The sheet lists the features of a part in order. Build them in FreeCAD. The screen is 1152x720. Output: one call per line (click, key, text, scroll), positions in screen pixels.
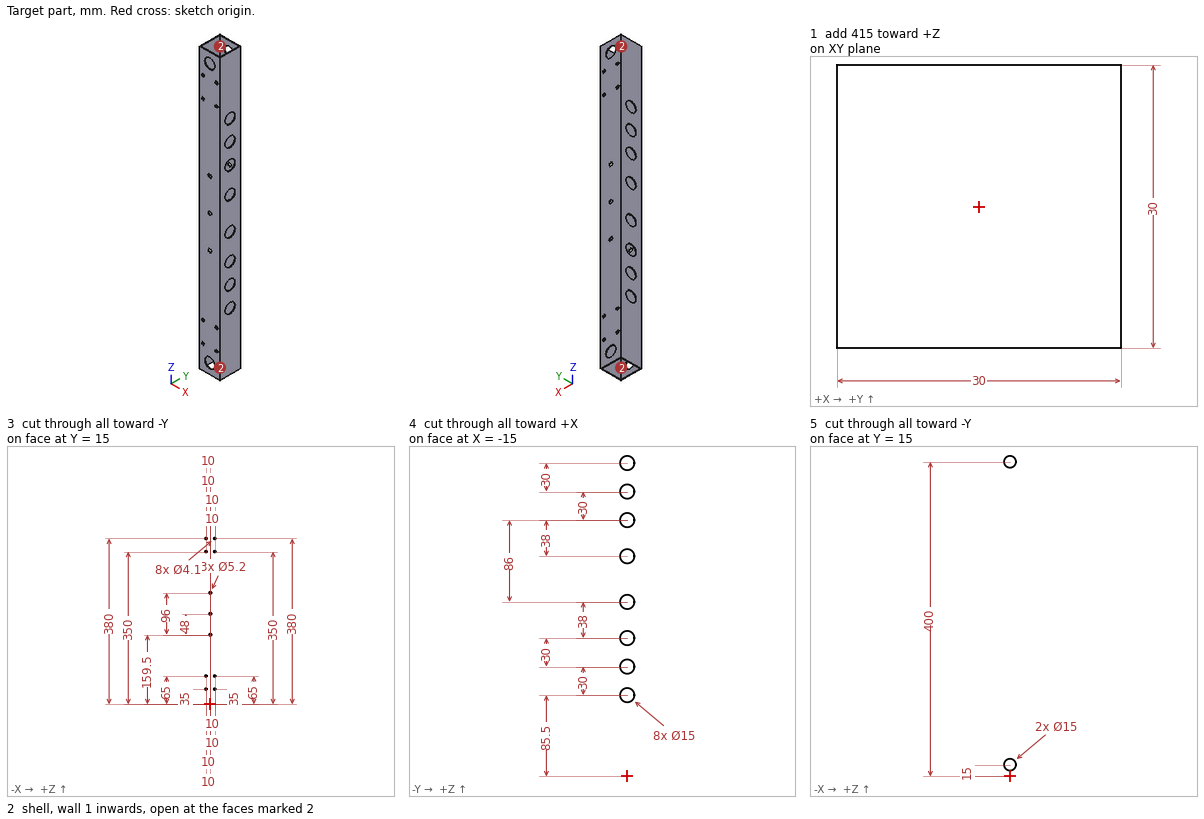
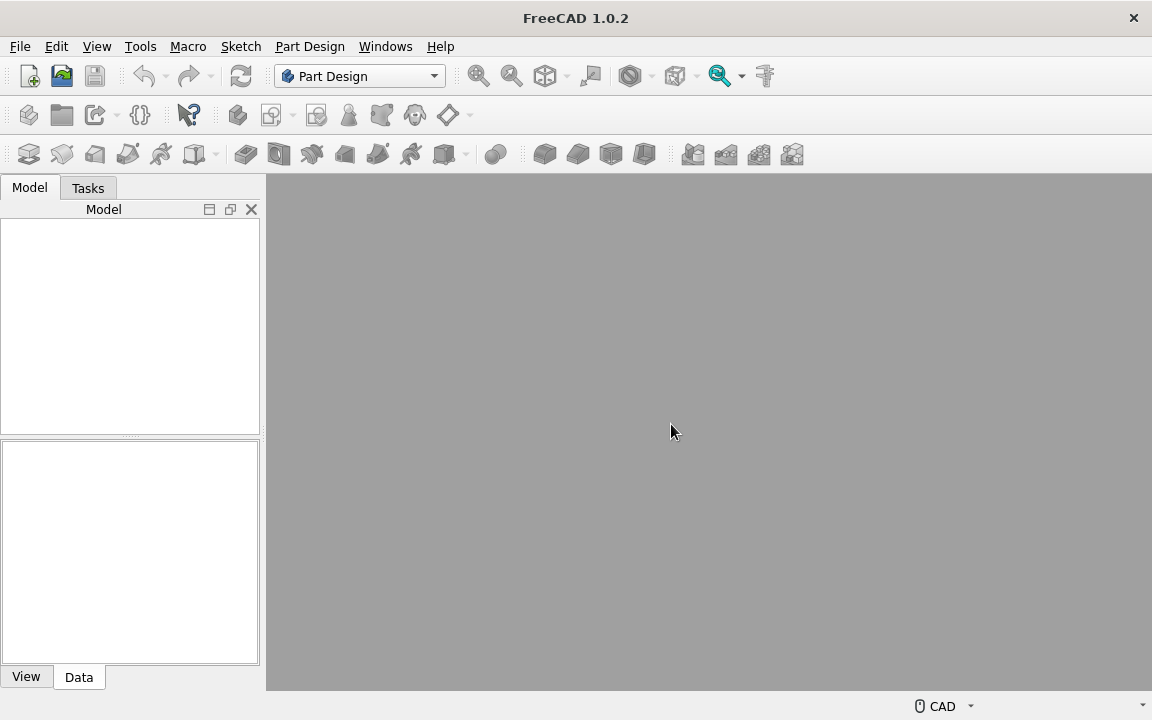
key(ctrl+n)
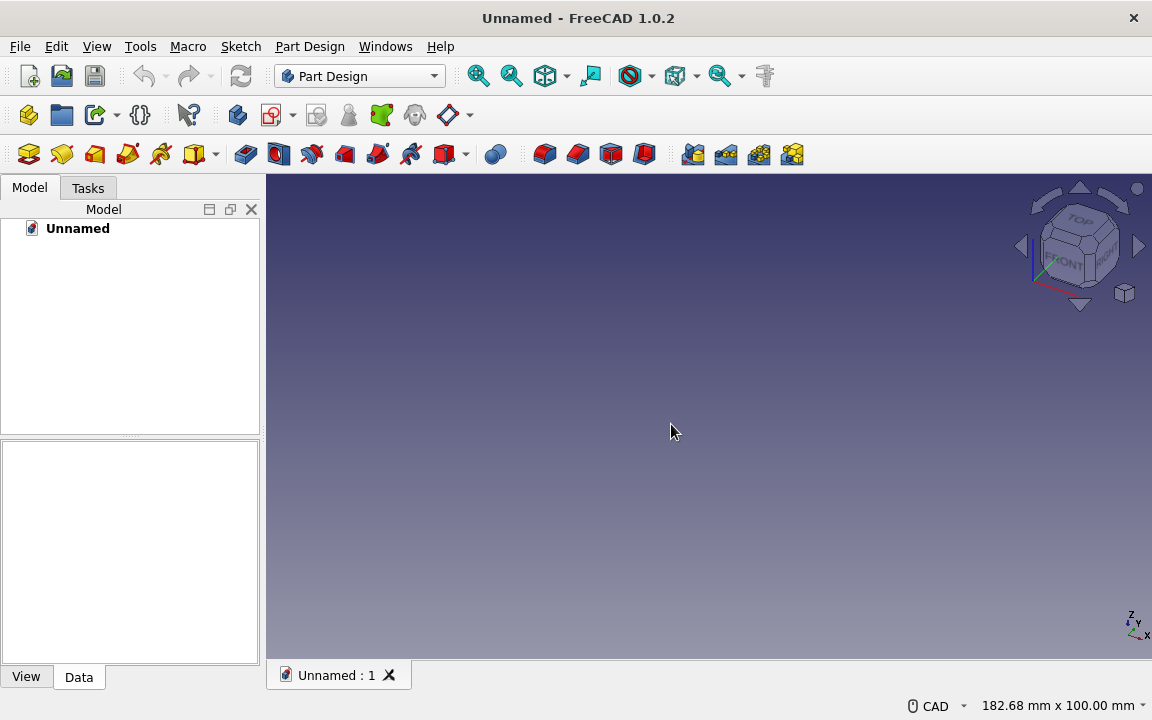
click(270, 116)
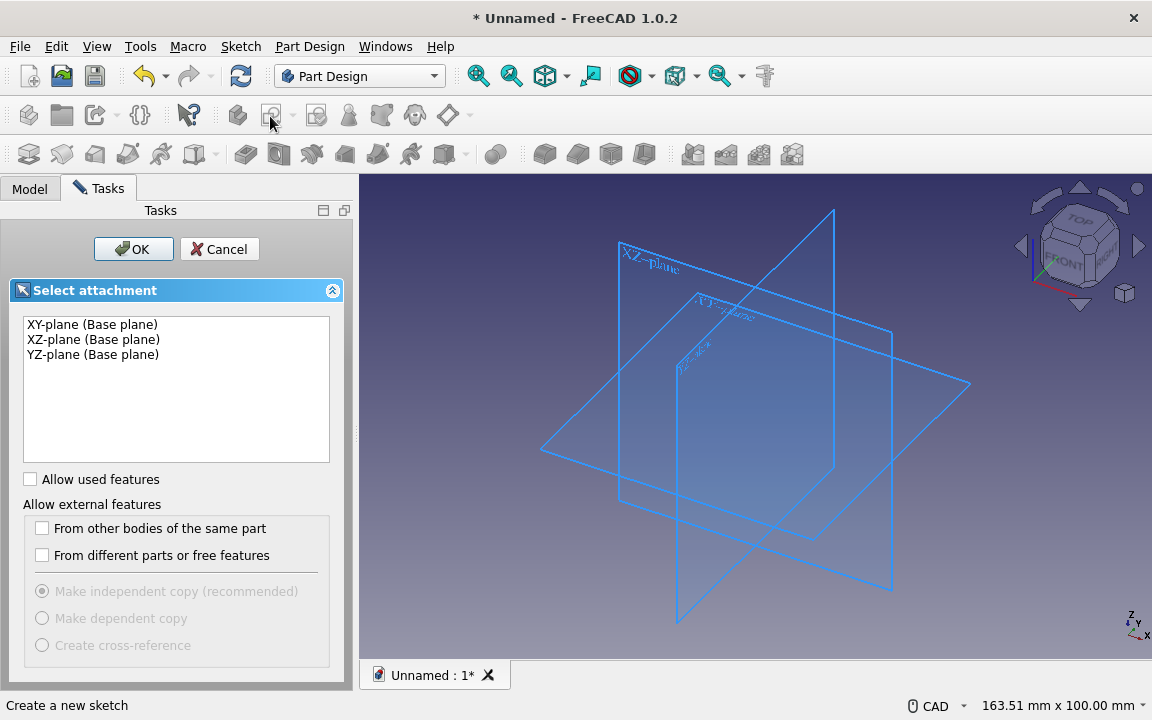
click(84, 324)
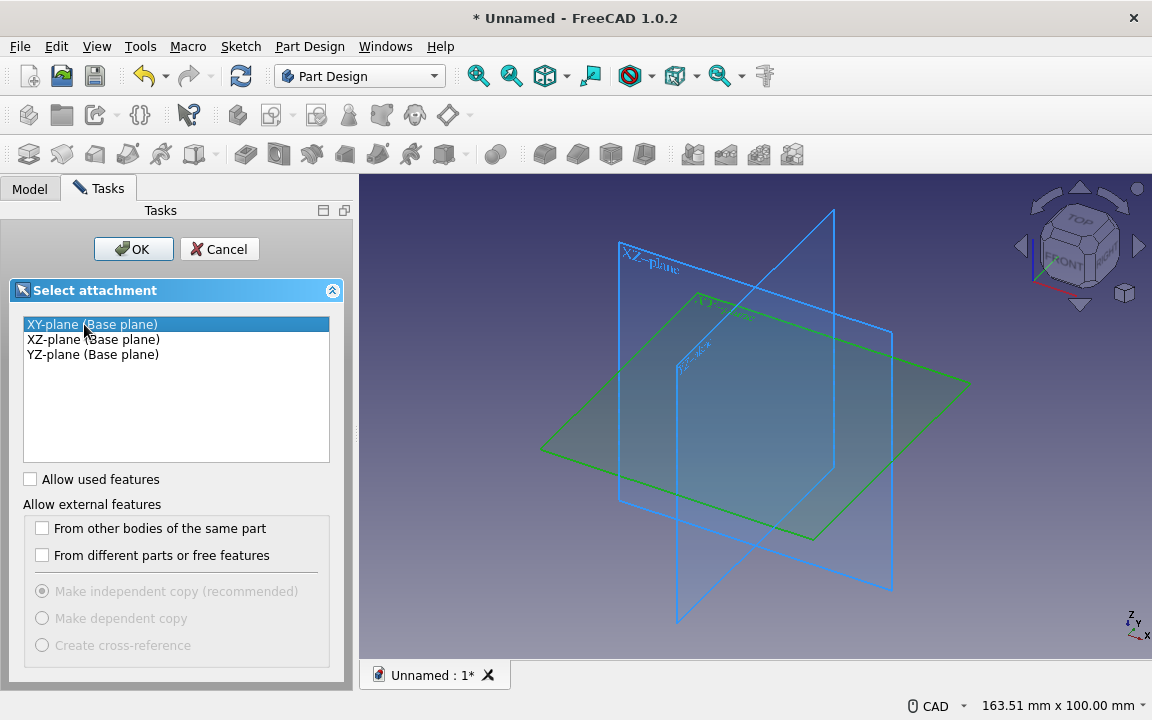
click(134, 249)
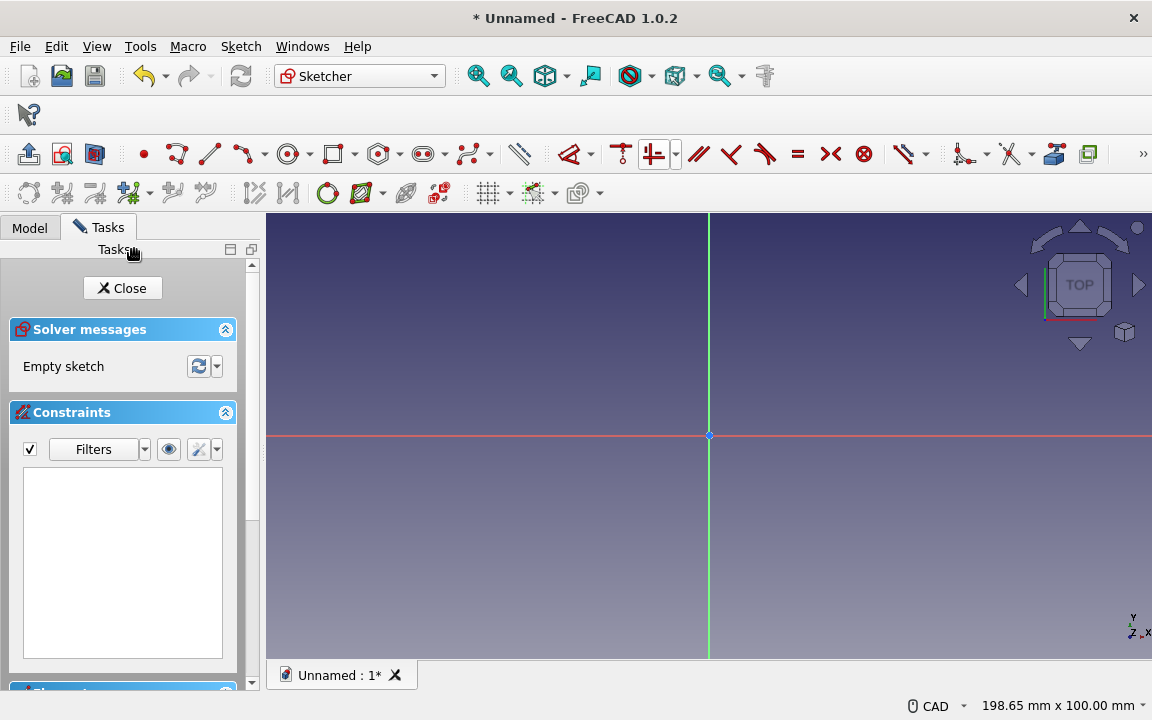
scroll(765, 436, up, 4)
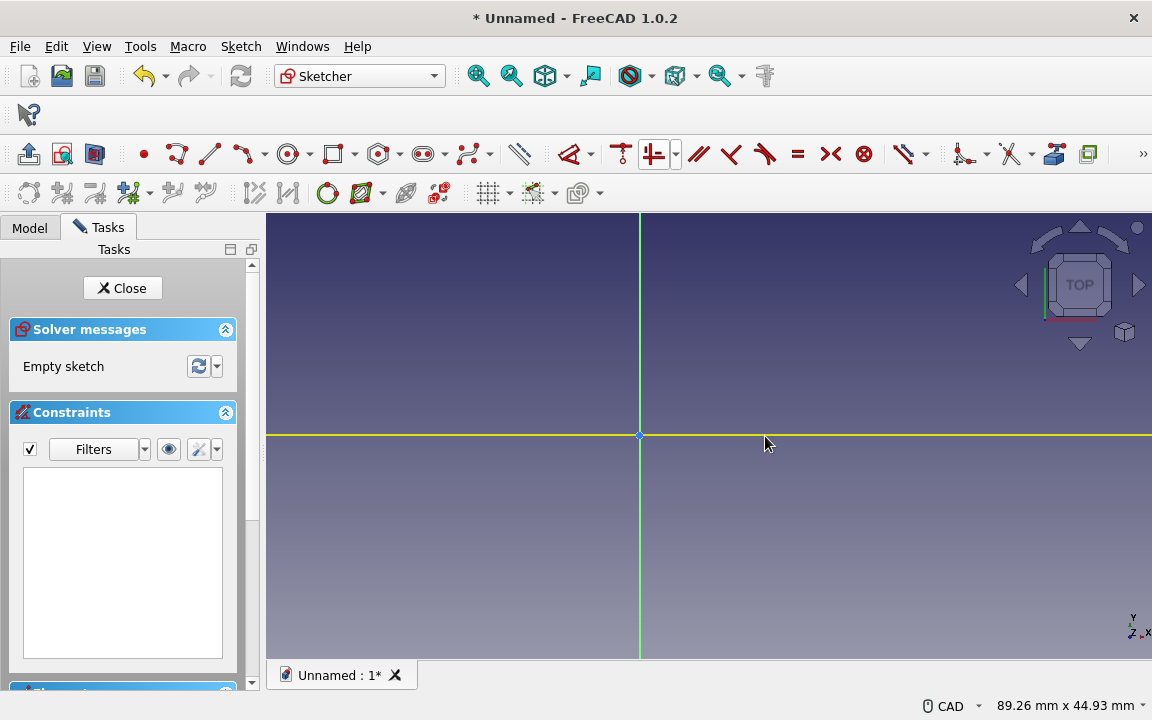
key(g)
key(v)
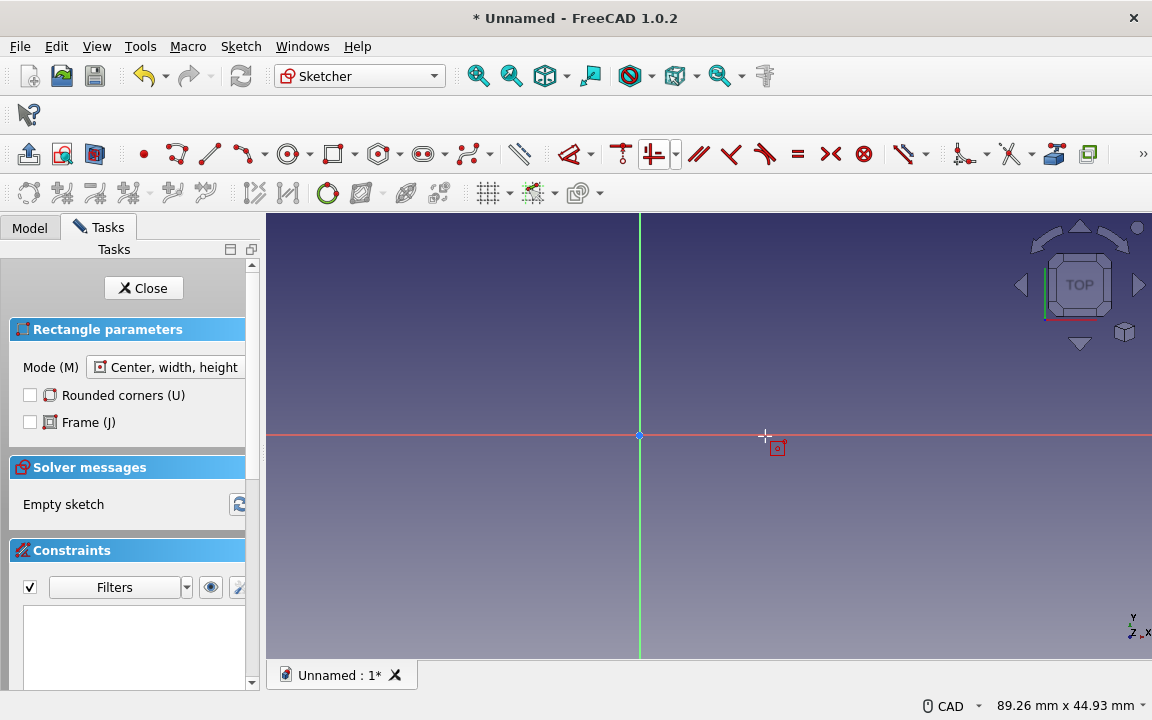
click(640, 435)
click(789, 286)
key(Escape)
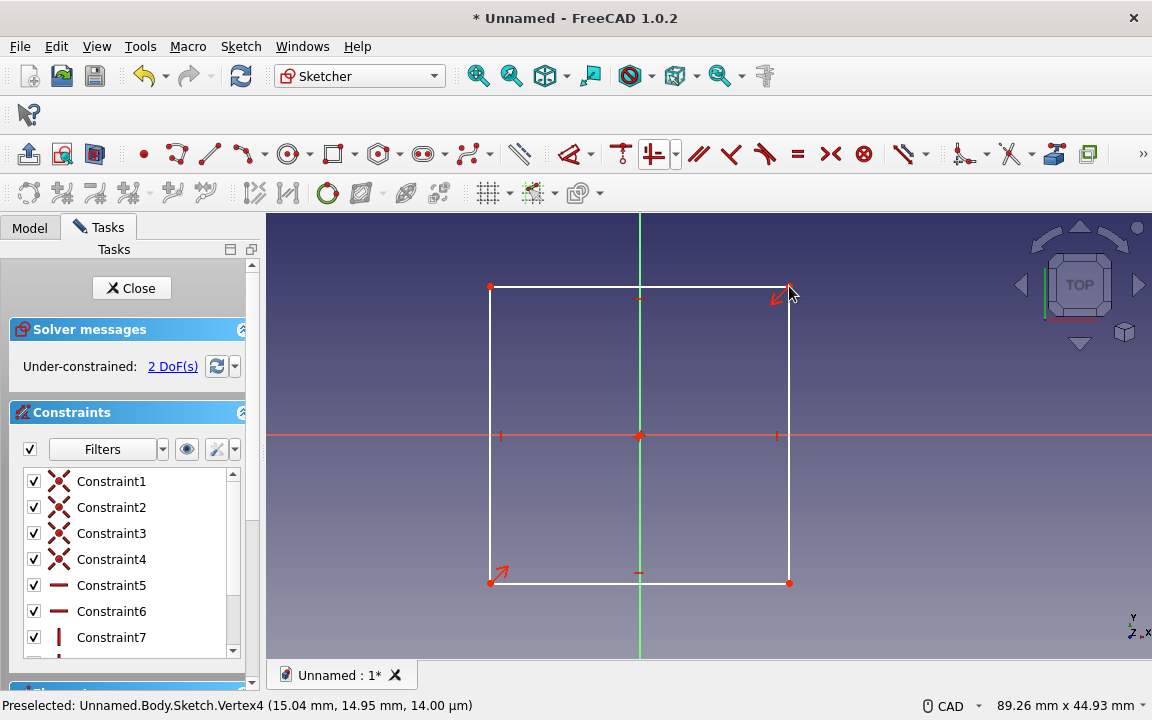
key(d)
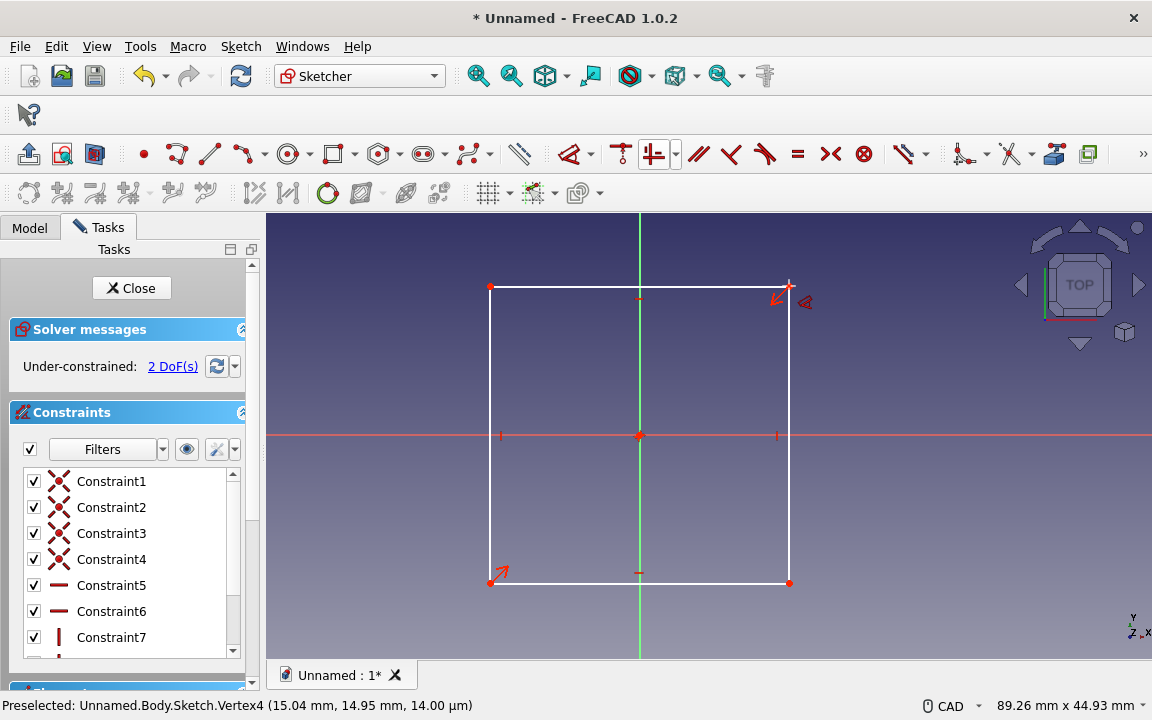
click(580, 584)
click(571, 618)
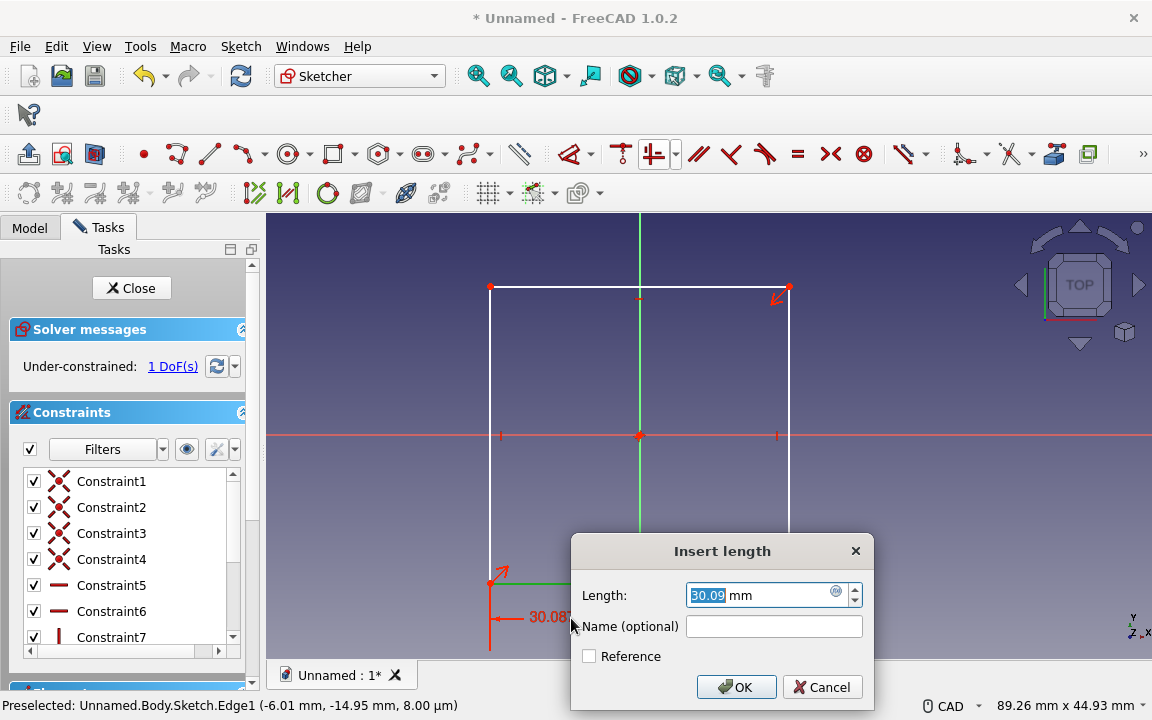
text(30)
key(Return)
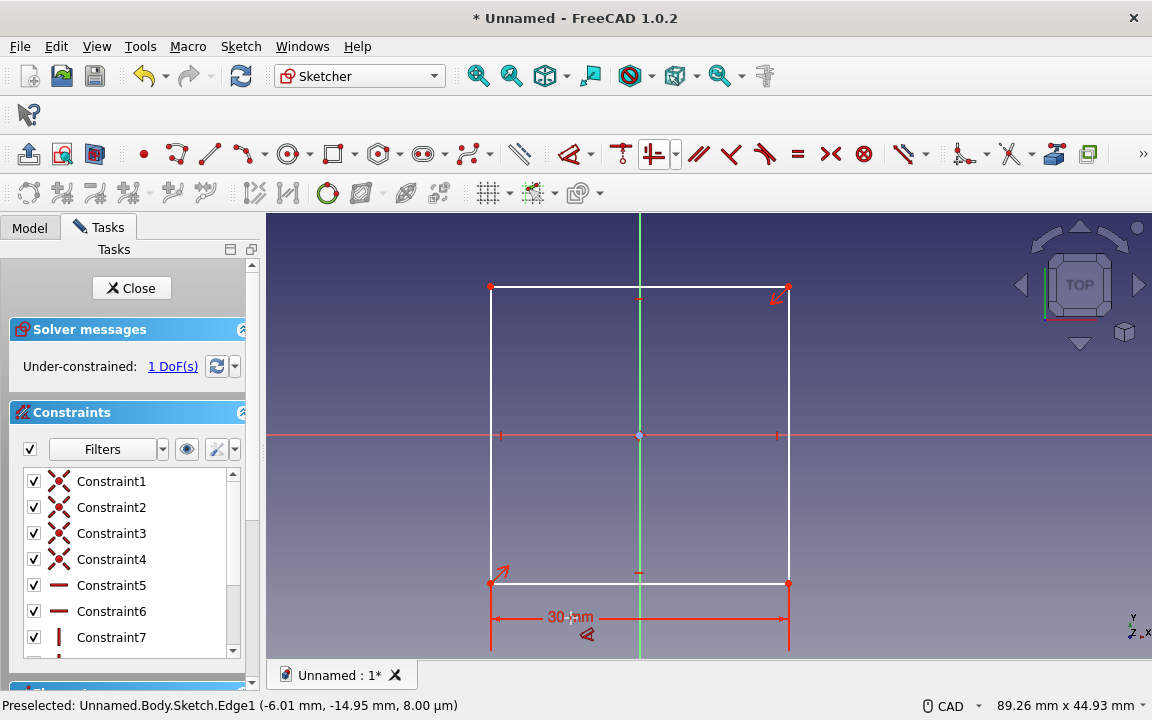
click(789, 495)
click(823, 367)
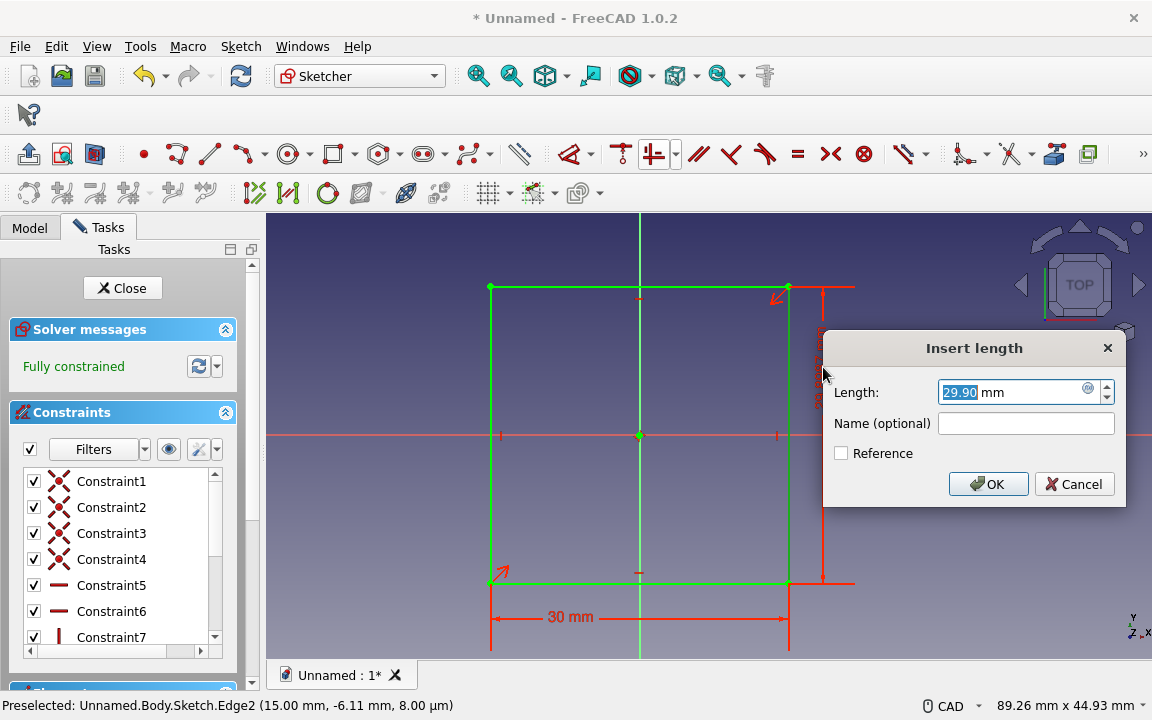
text(30)
key(Return)
key(Escape)